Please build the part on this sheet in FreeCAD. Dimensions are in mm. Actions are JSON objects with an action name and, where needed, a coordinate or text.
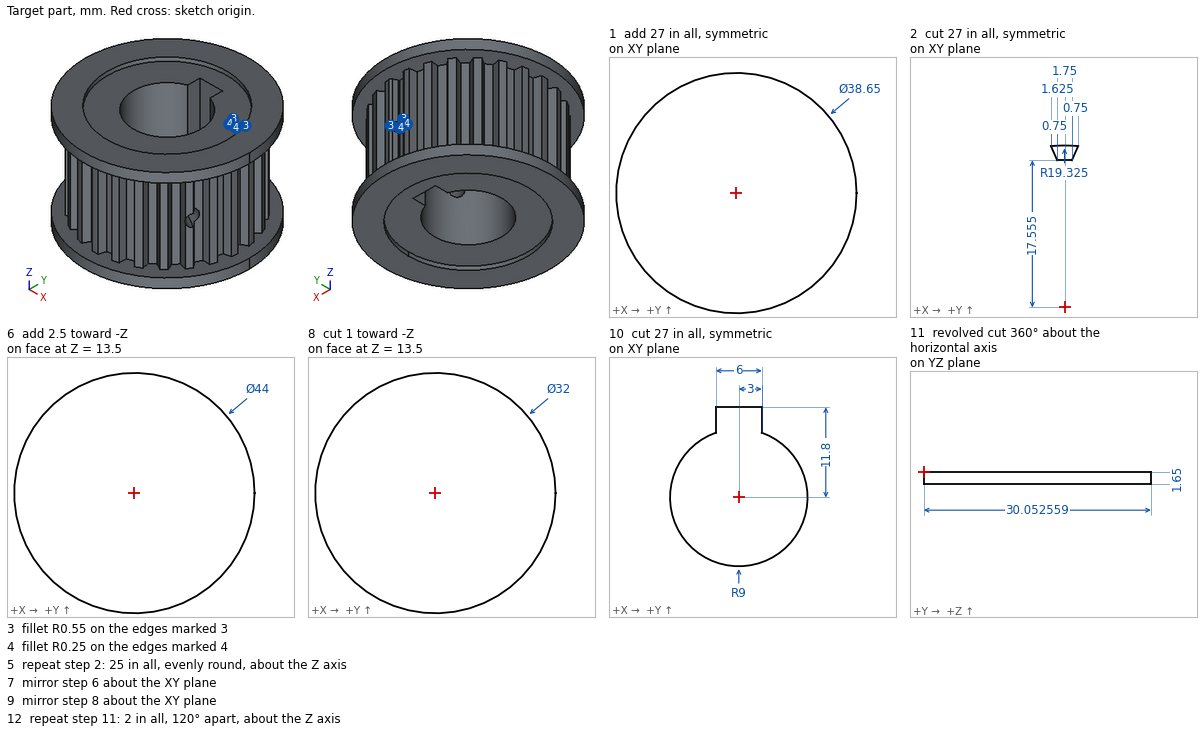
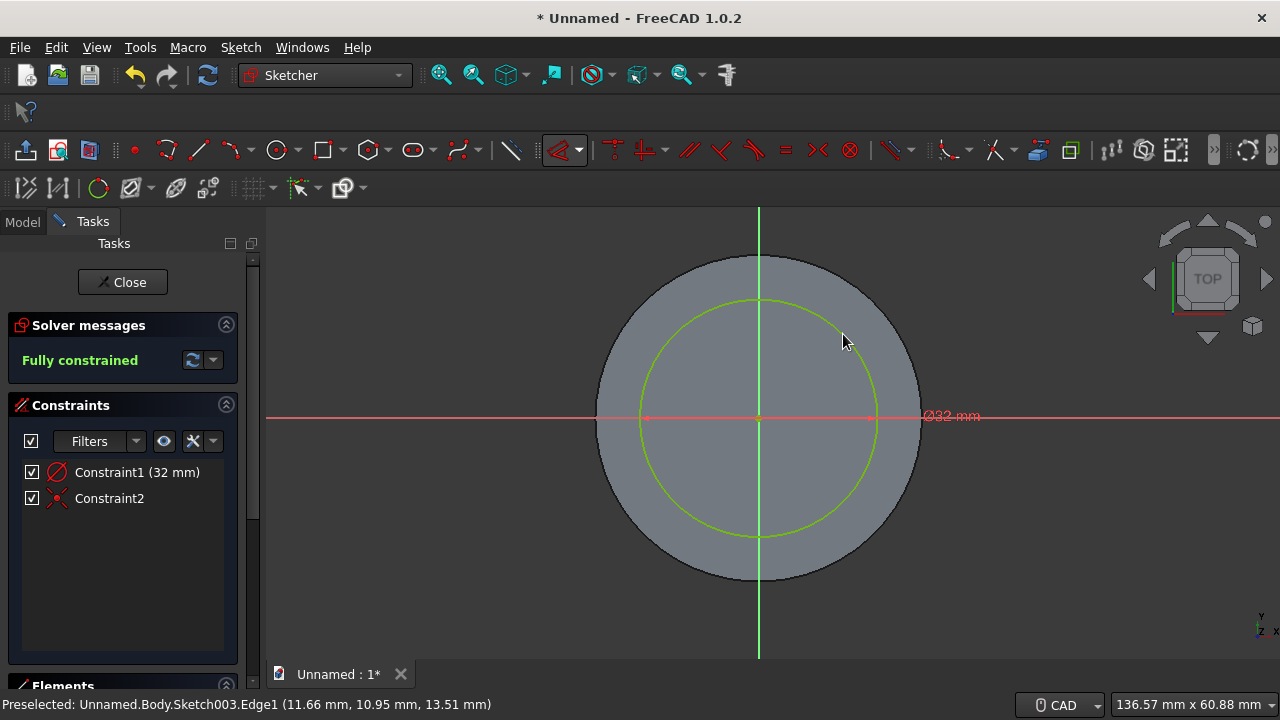
{"action": "left_click", "coordinate": [123, 282]}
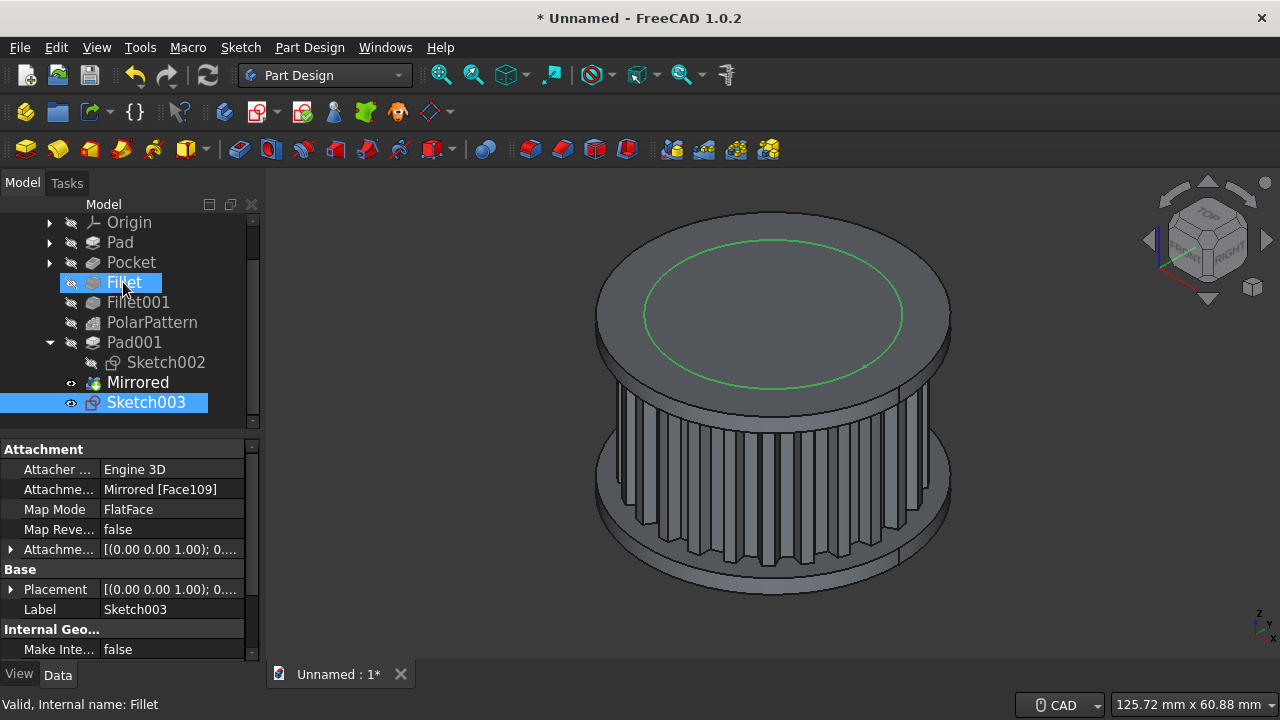
{"action": "left_click", "coordinate": [240, 150]}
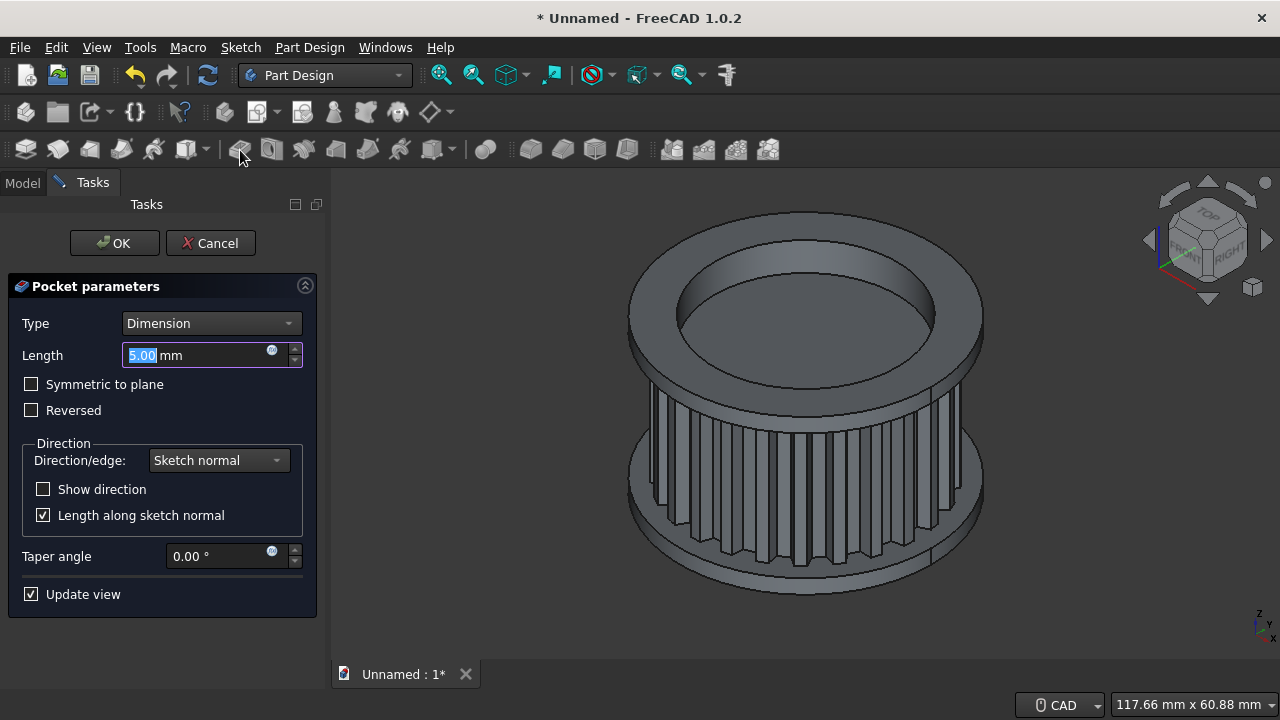
{"action": "type", "text": "1"}
{"action": "key", "text": "Tab"}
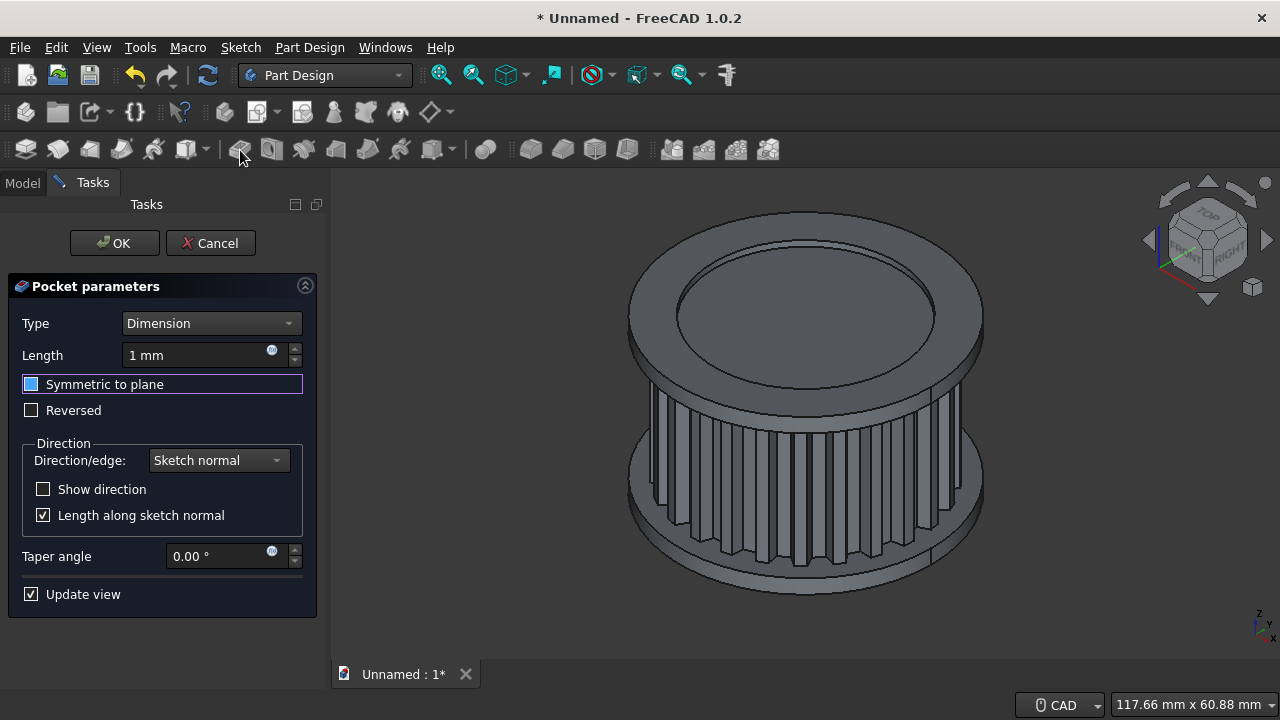
{"action": "left_click", "coordinate": [115, 243]}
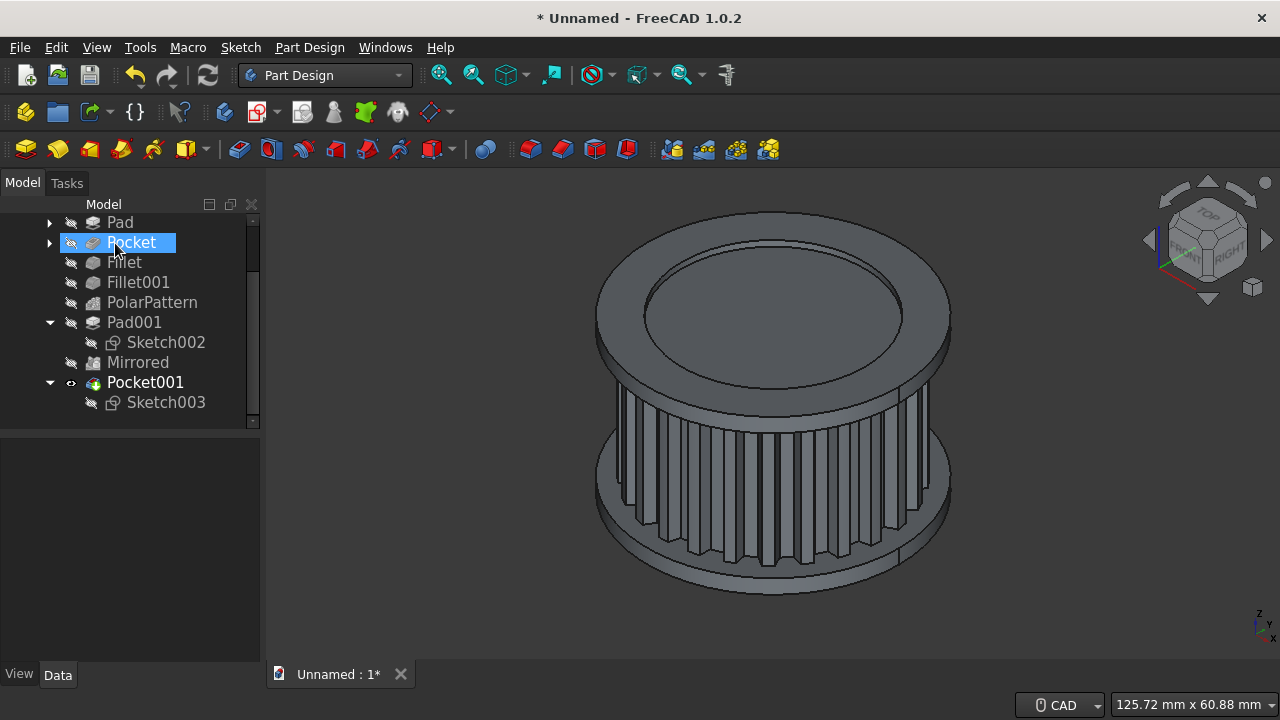
{"action": "left_click", "coordinate": [116, 383]}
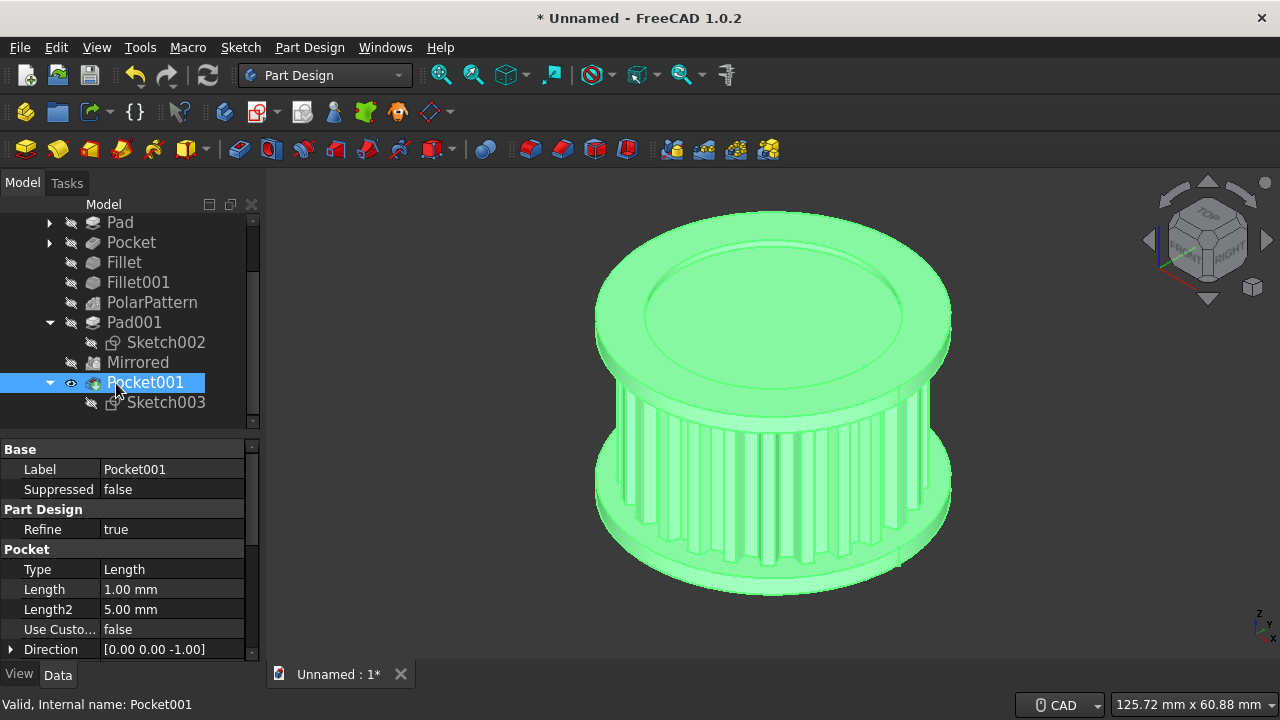
{"action": "left_click", "coordinate": [672, 150]}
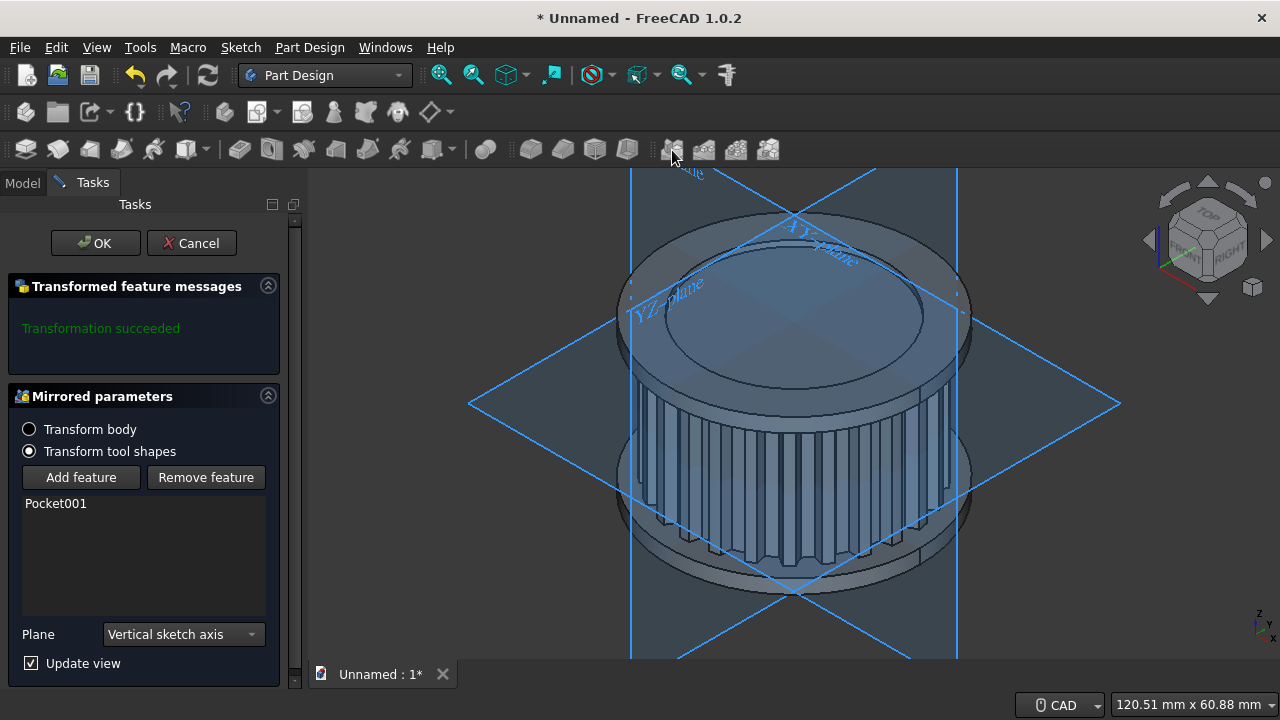
{"action": "left_click", "coordinate": [184, 634]}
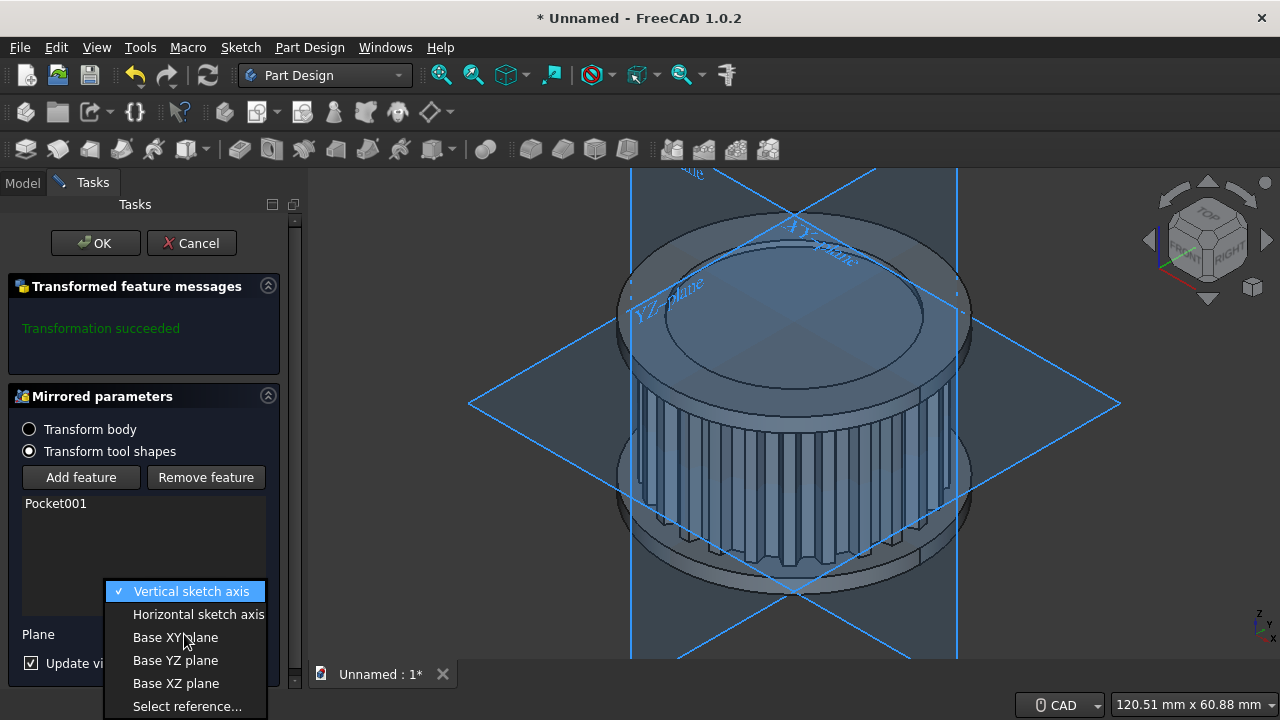
{"action": "left_click", "coordinate": [184, 638]}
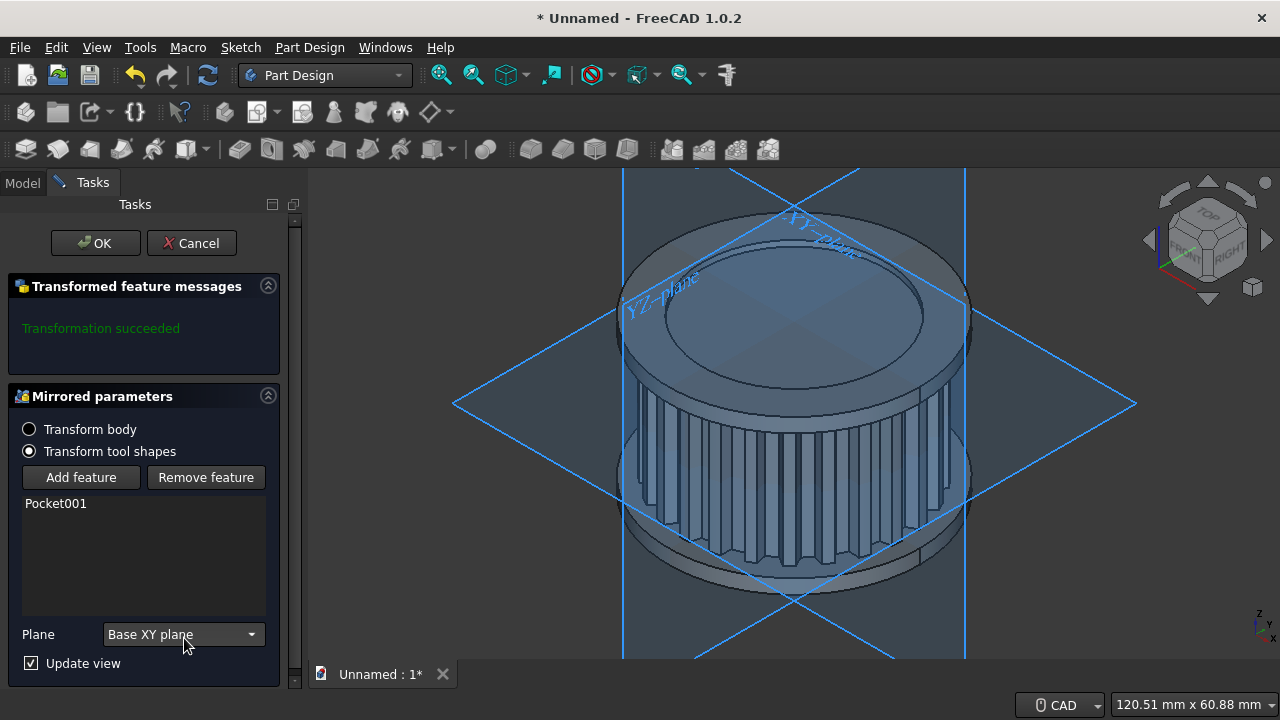
{"action": "left_click", "coordinate": [96, 243]}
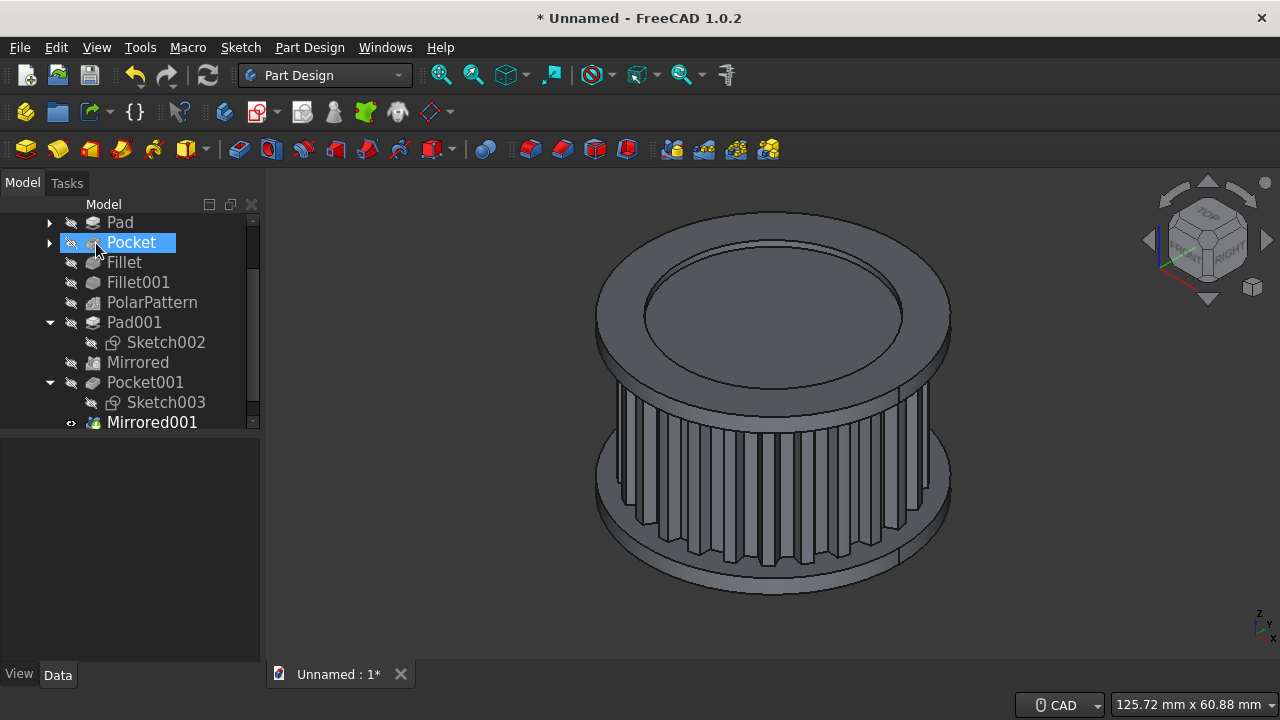
{"action": "left_click", "coordinate": [258, 112]}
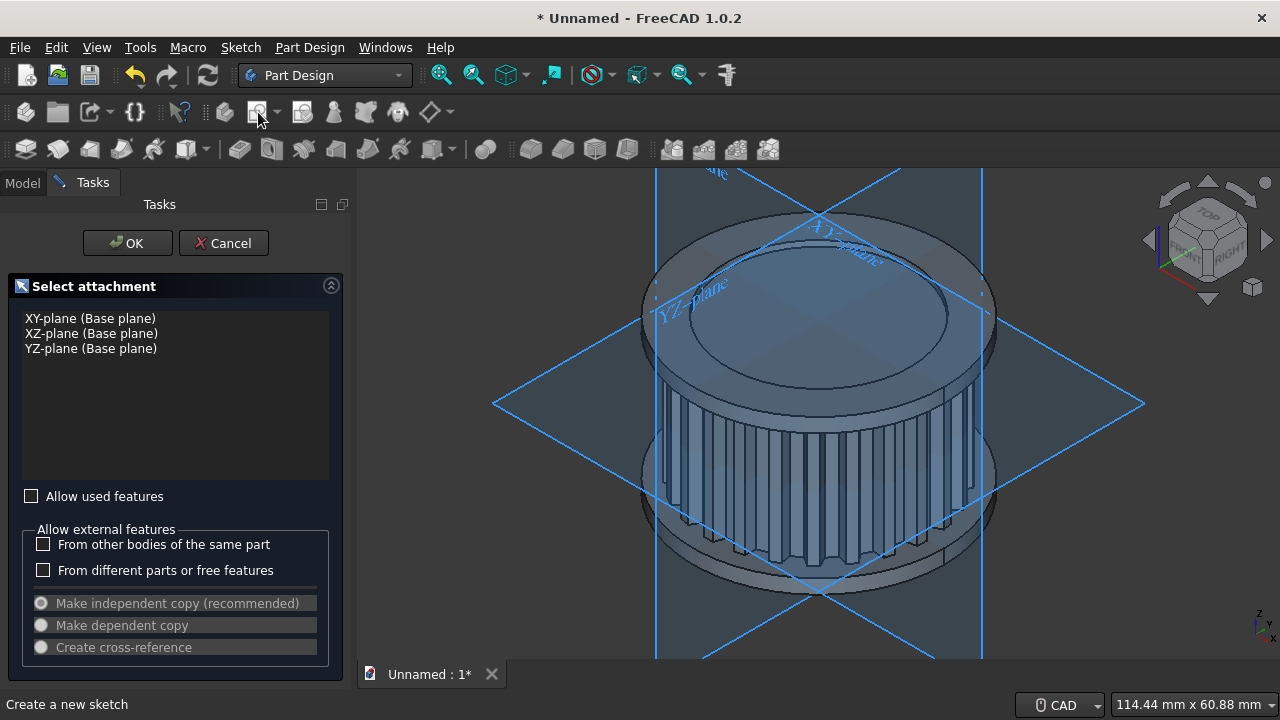
{"action": "left_click", "coordinate": [82, 318]}